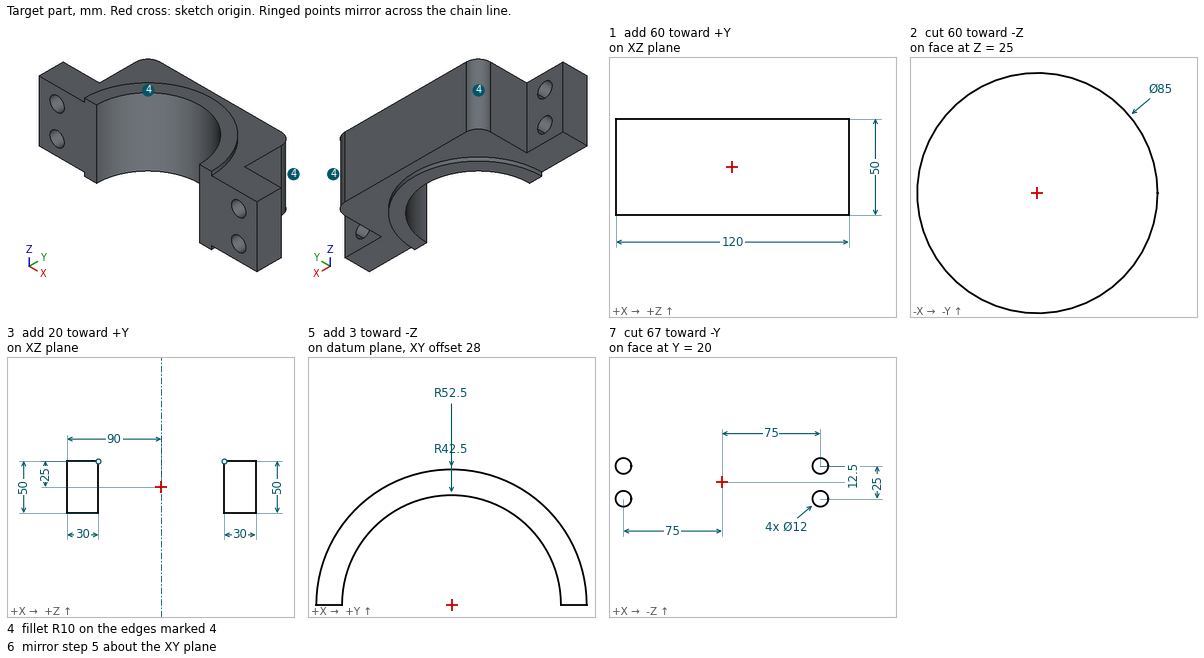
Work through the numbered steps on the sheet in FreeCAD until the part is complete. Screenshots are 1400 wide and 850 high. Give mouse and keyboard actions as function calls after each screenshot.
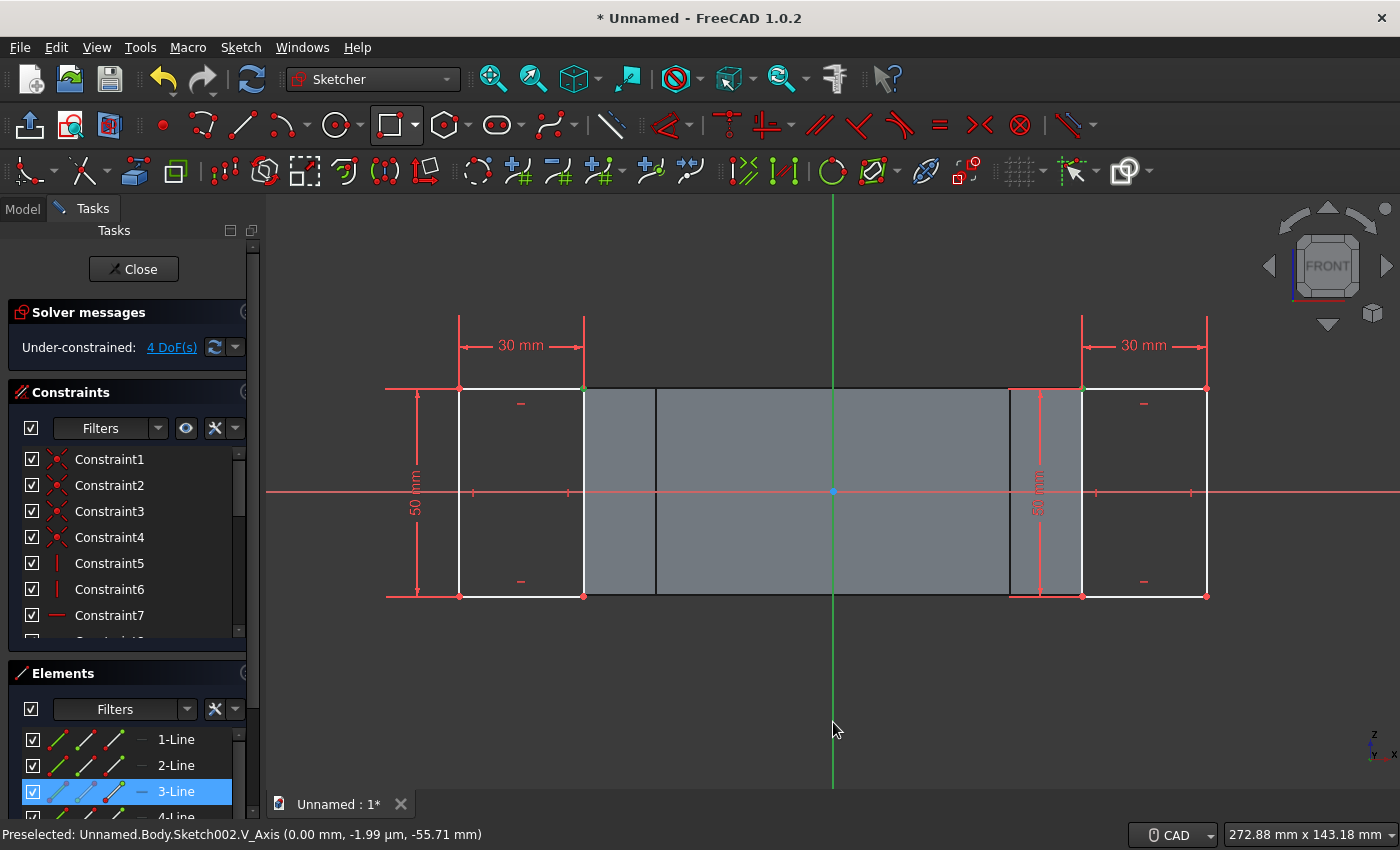
click(980, 126)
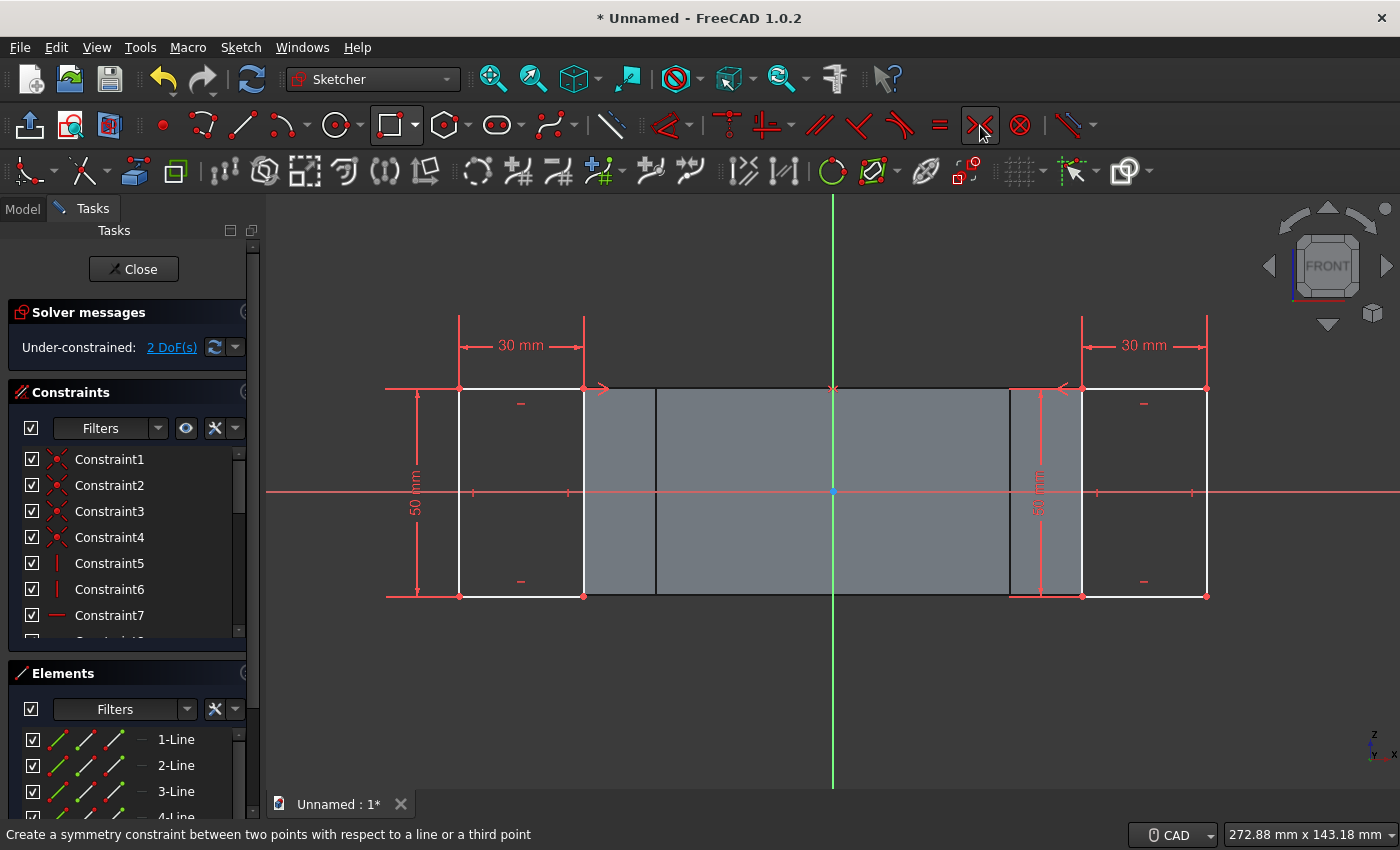
click(666, 126)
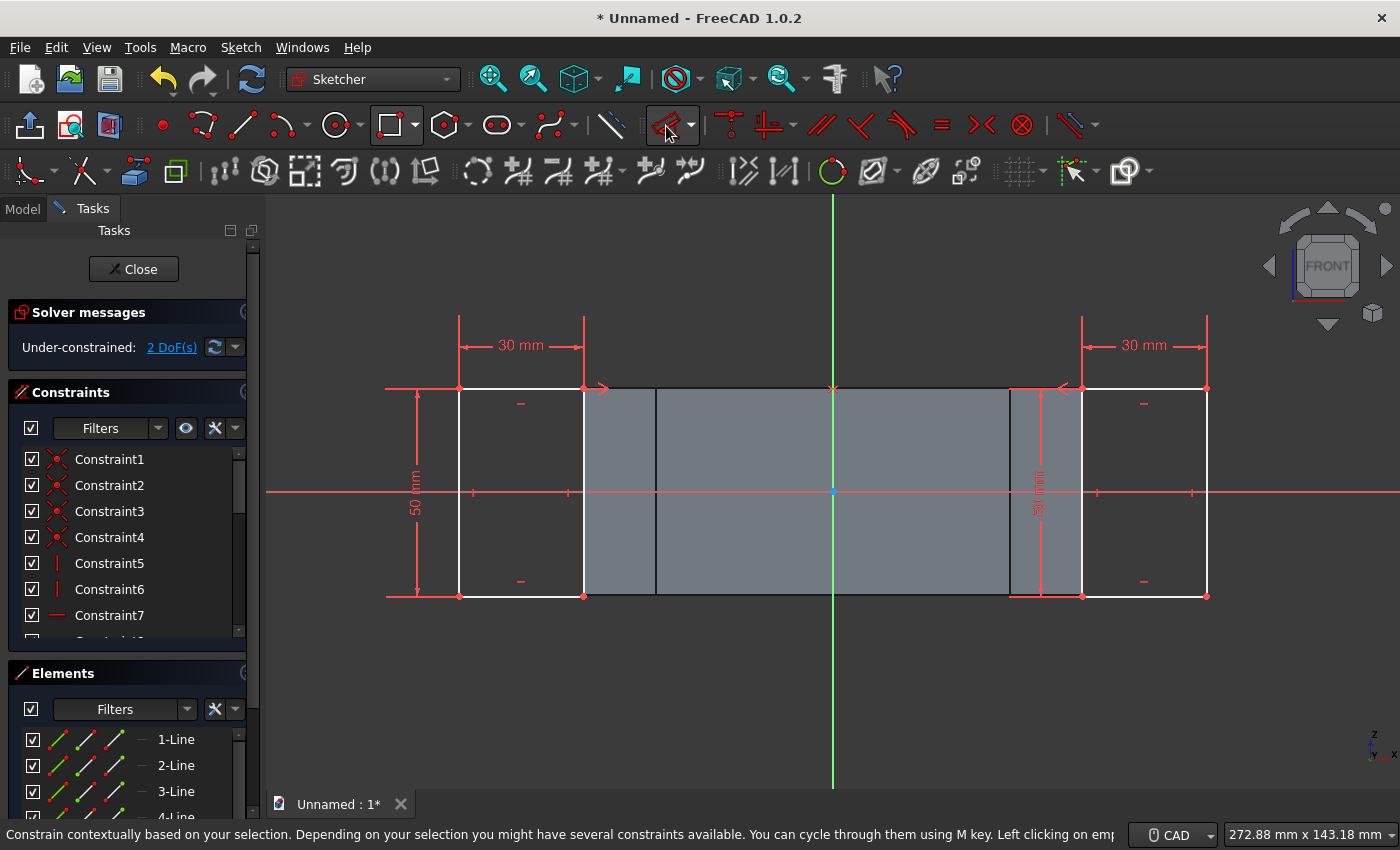
click(459, 389)
click(646, 355)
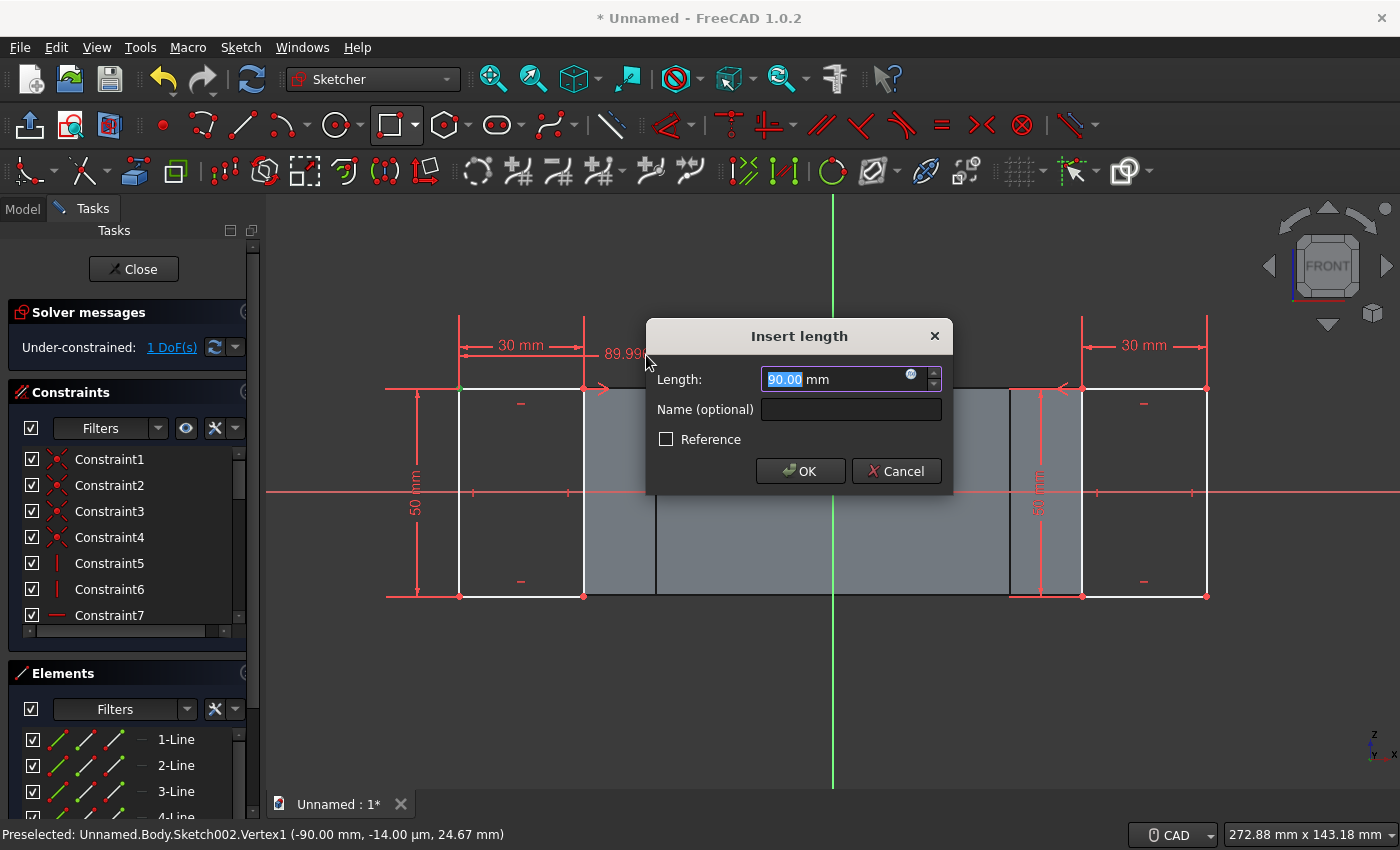
text(90)
key(Return)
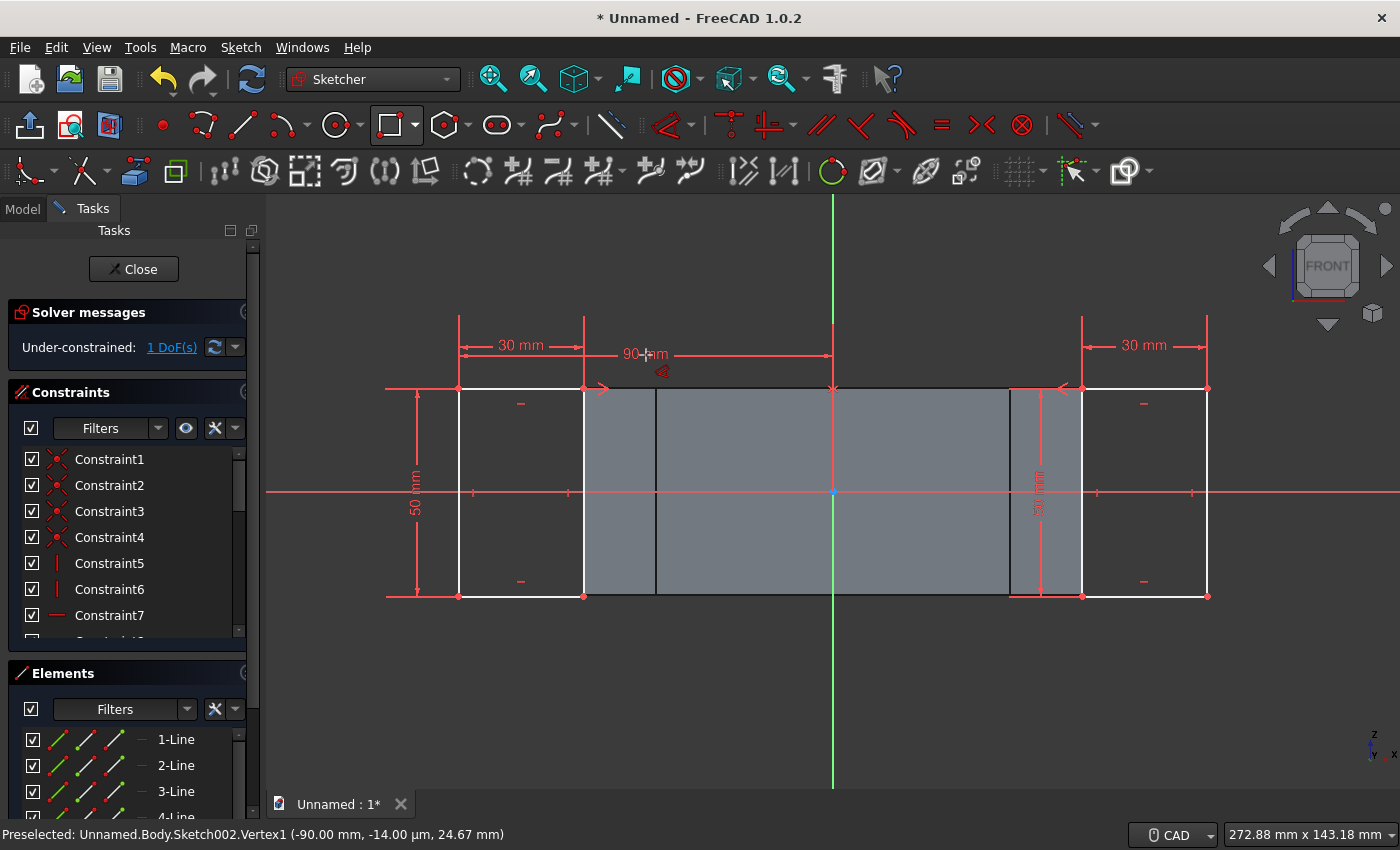
click(459, 389)
click(425, 440)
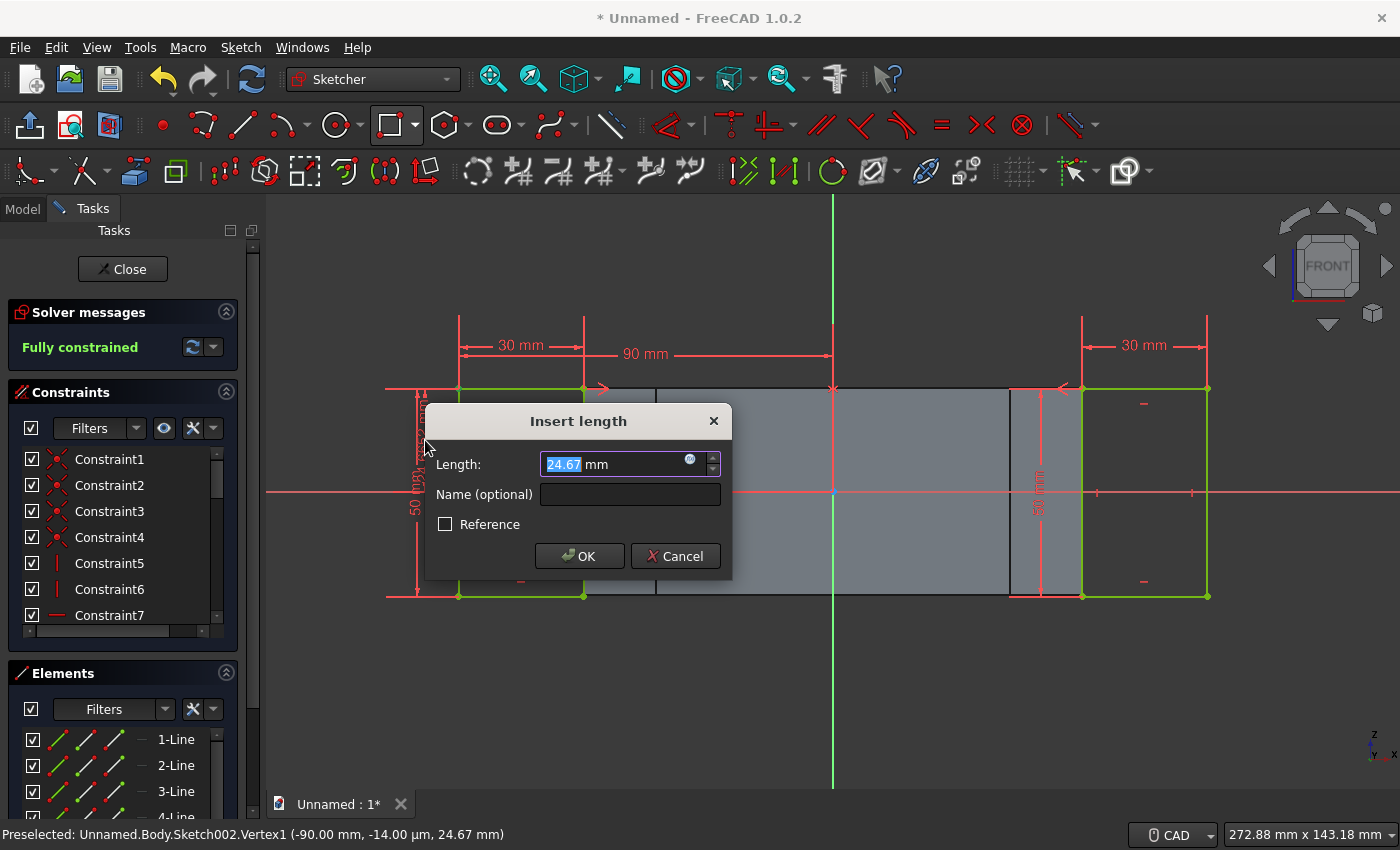
text(25)
key(Return)
key(Escape)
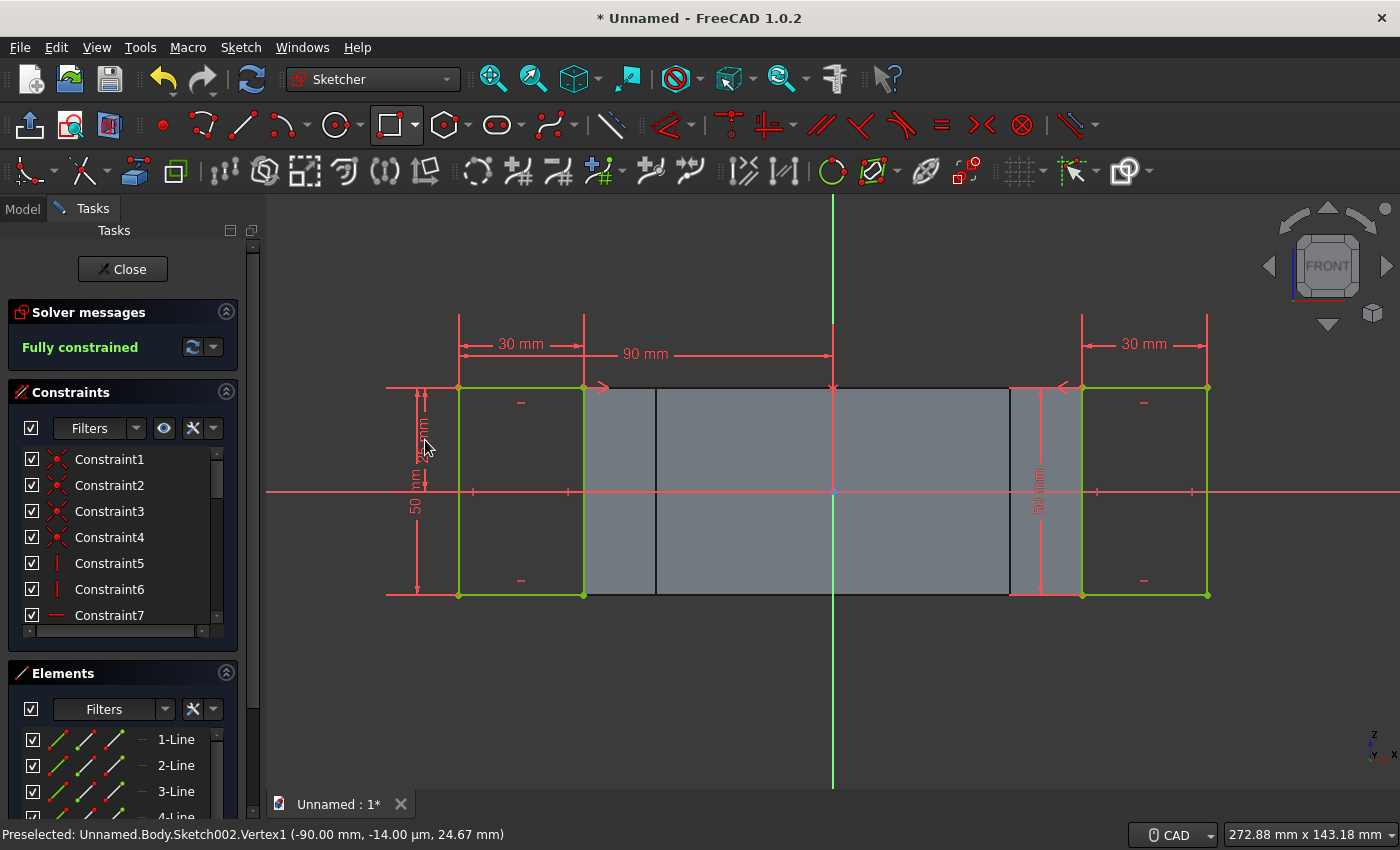
click(123, 269)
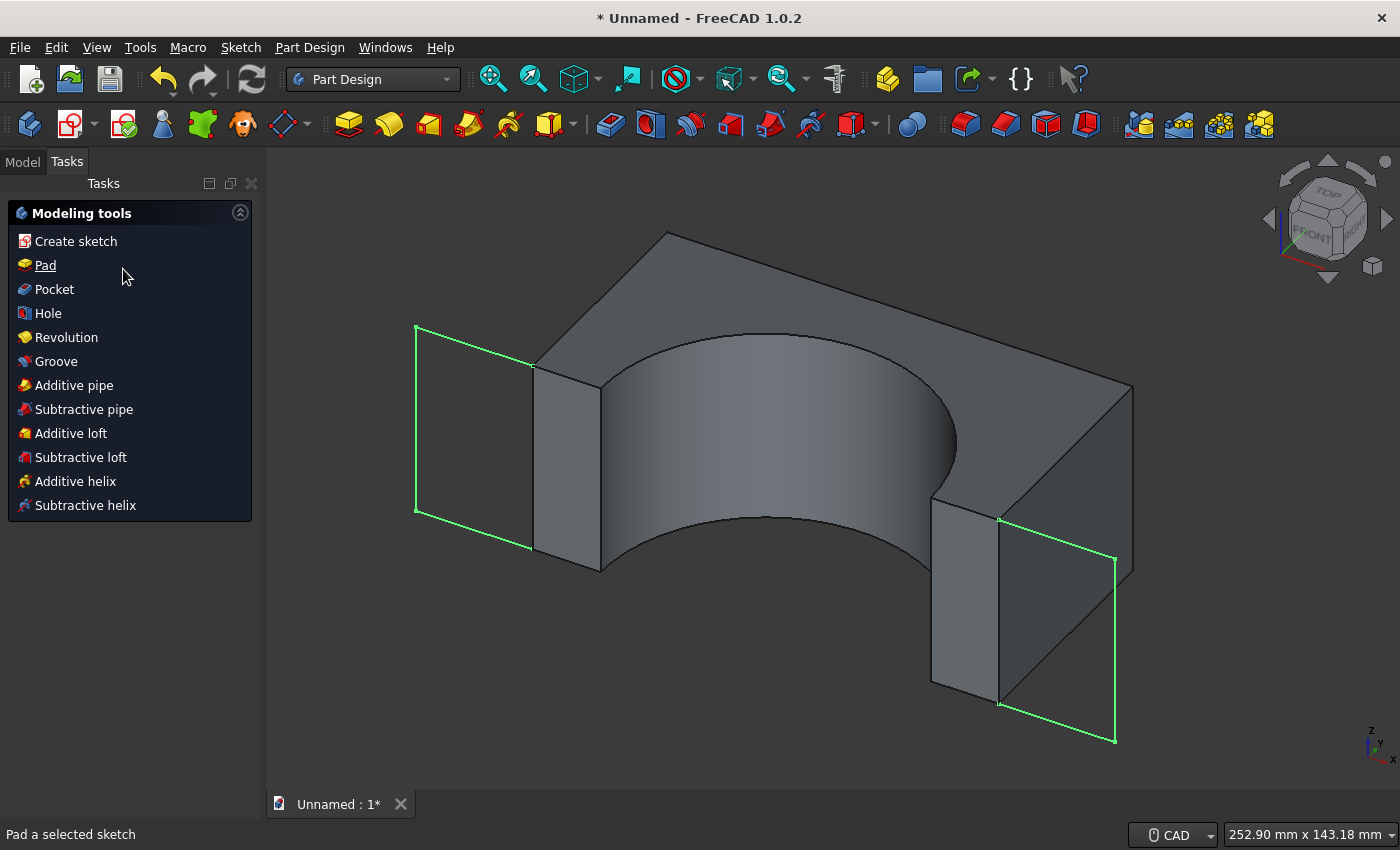
click(350, 124)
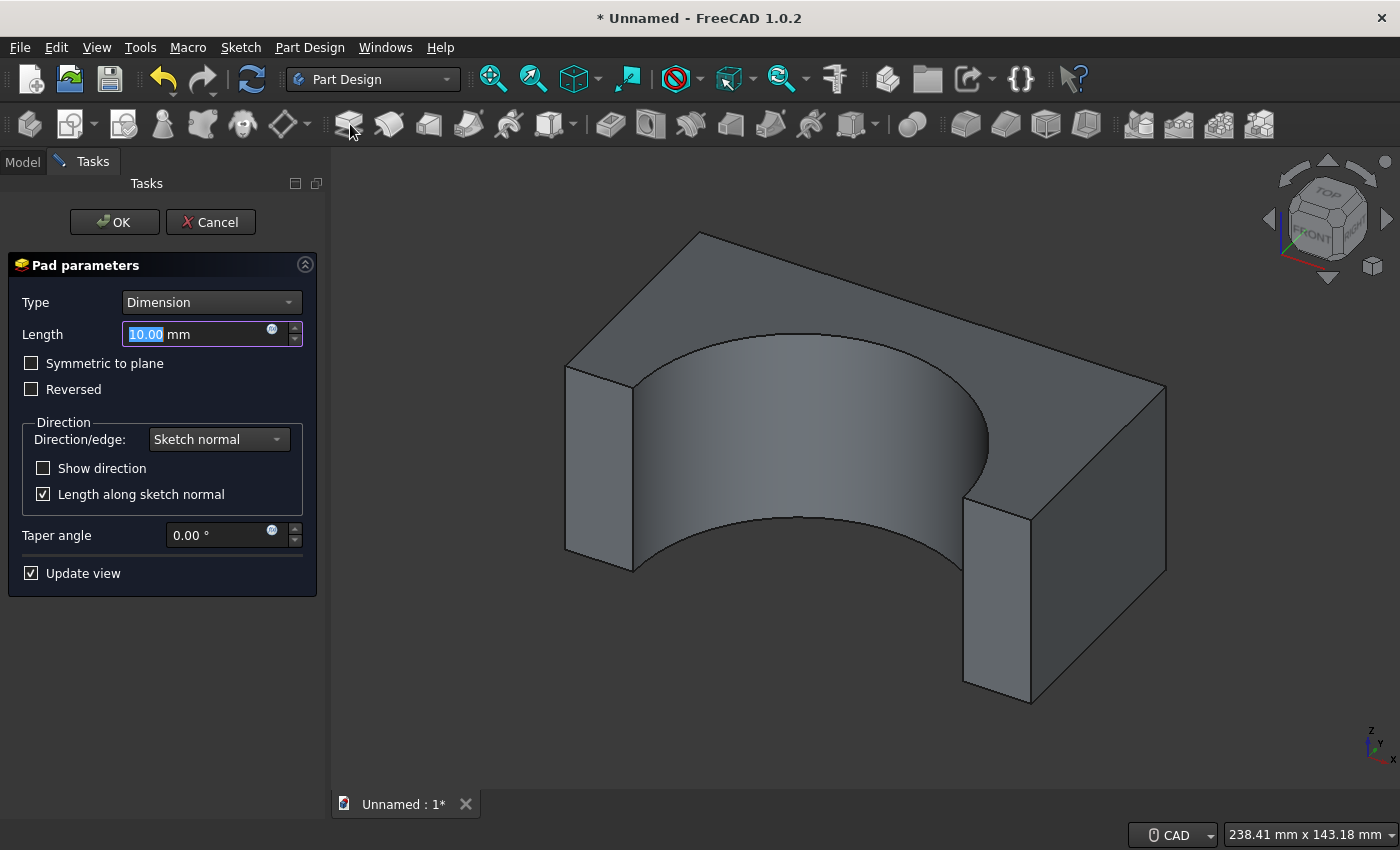
text(20)
key(Tab)